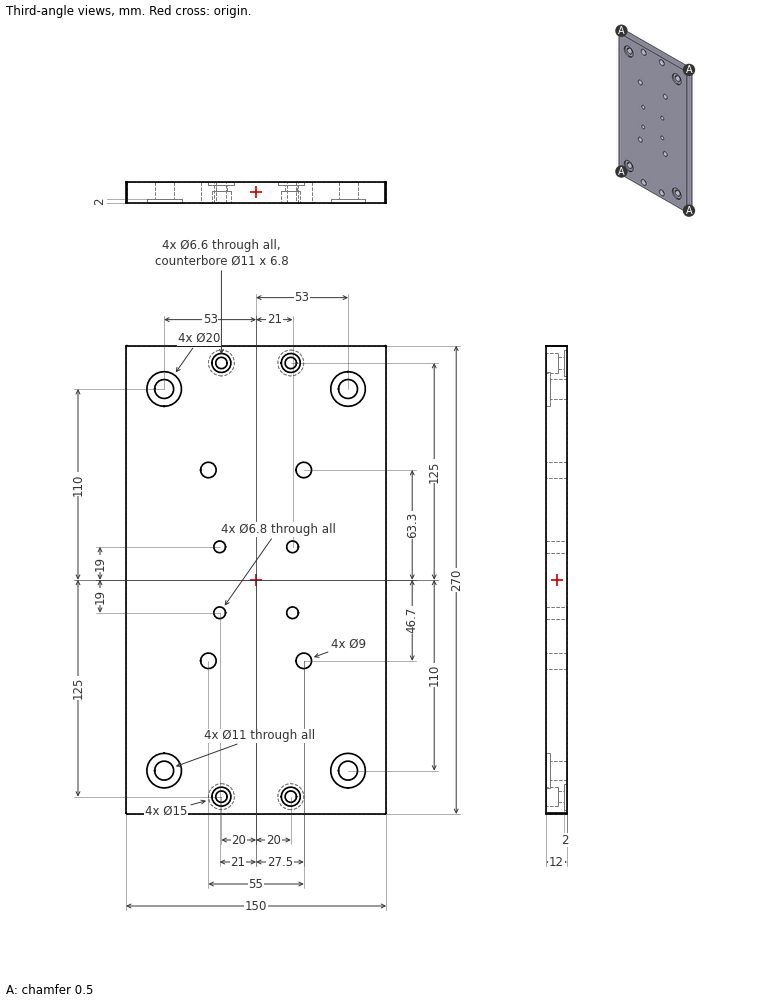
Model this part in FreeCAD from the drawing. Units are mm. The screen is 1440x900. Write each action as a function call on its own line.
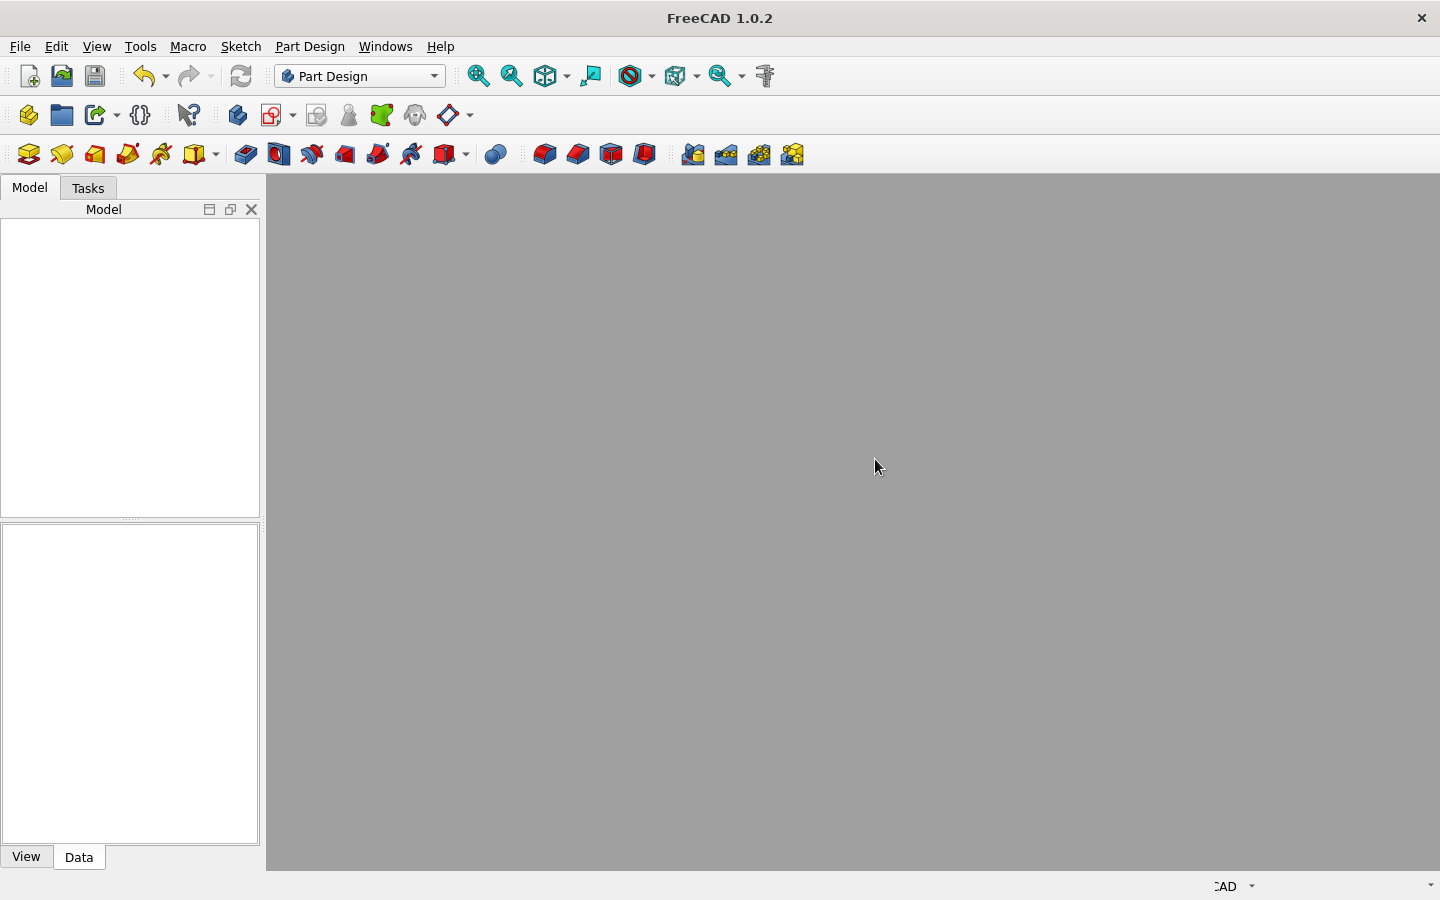
key(ctrl+n)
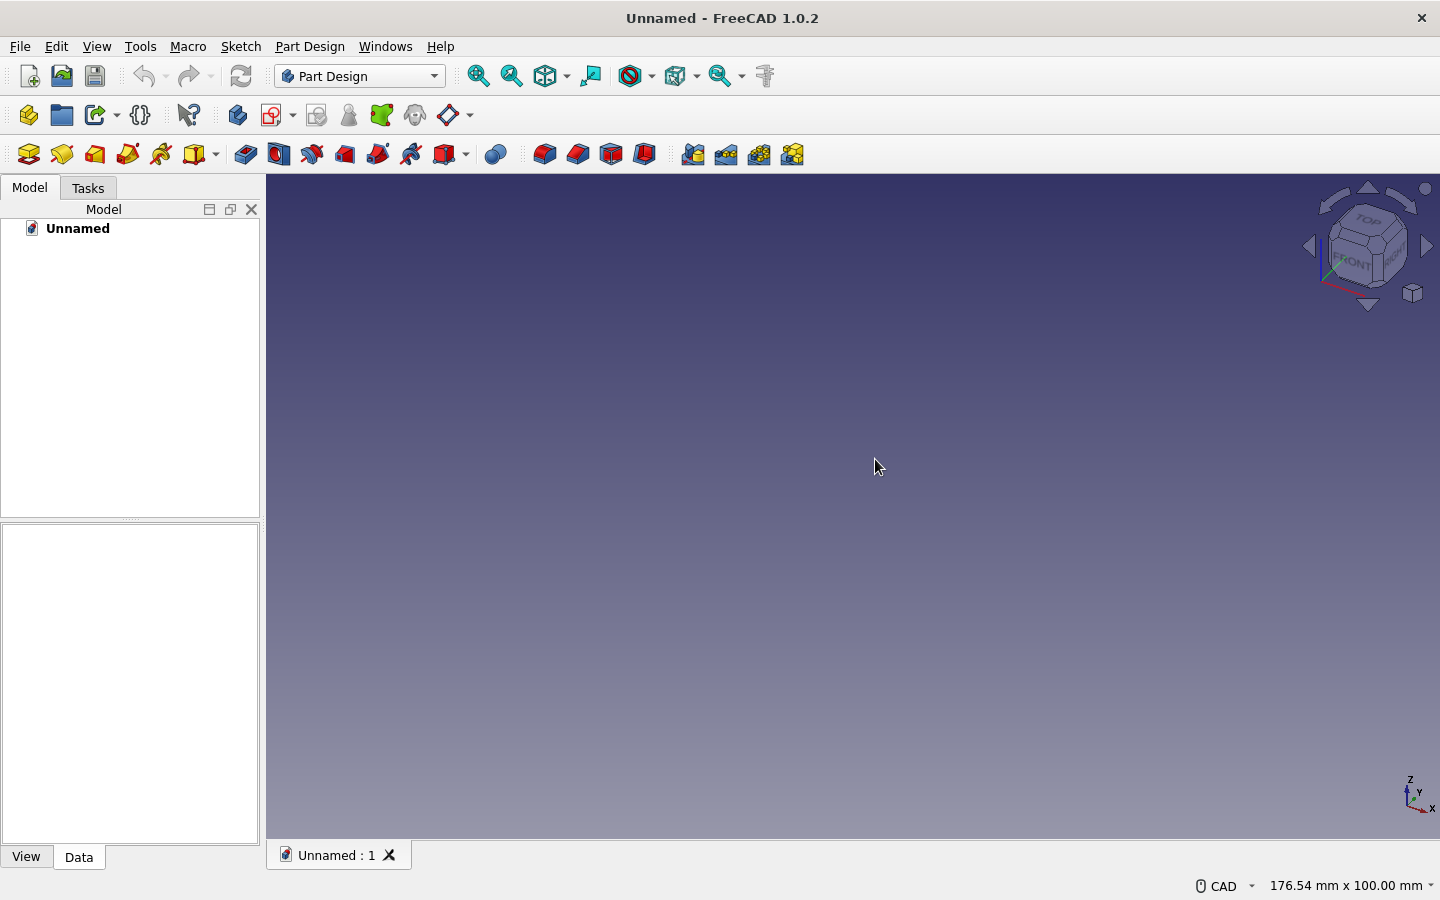
click(270, 116)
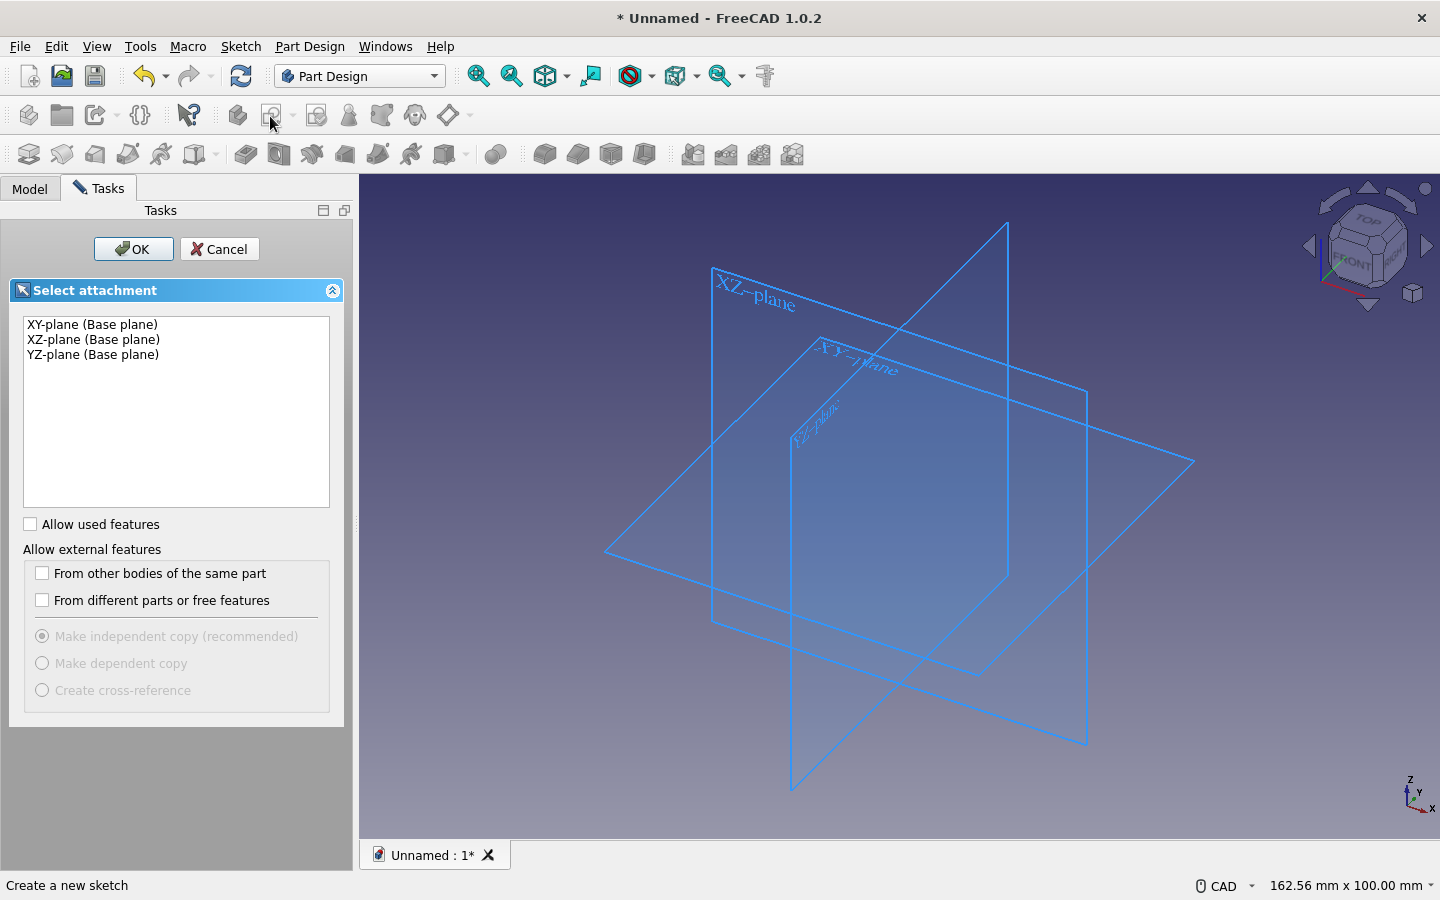
click(84, 340)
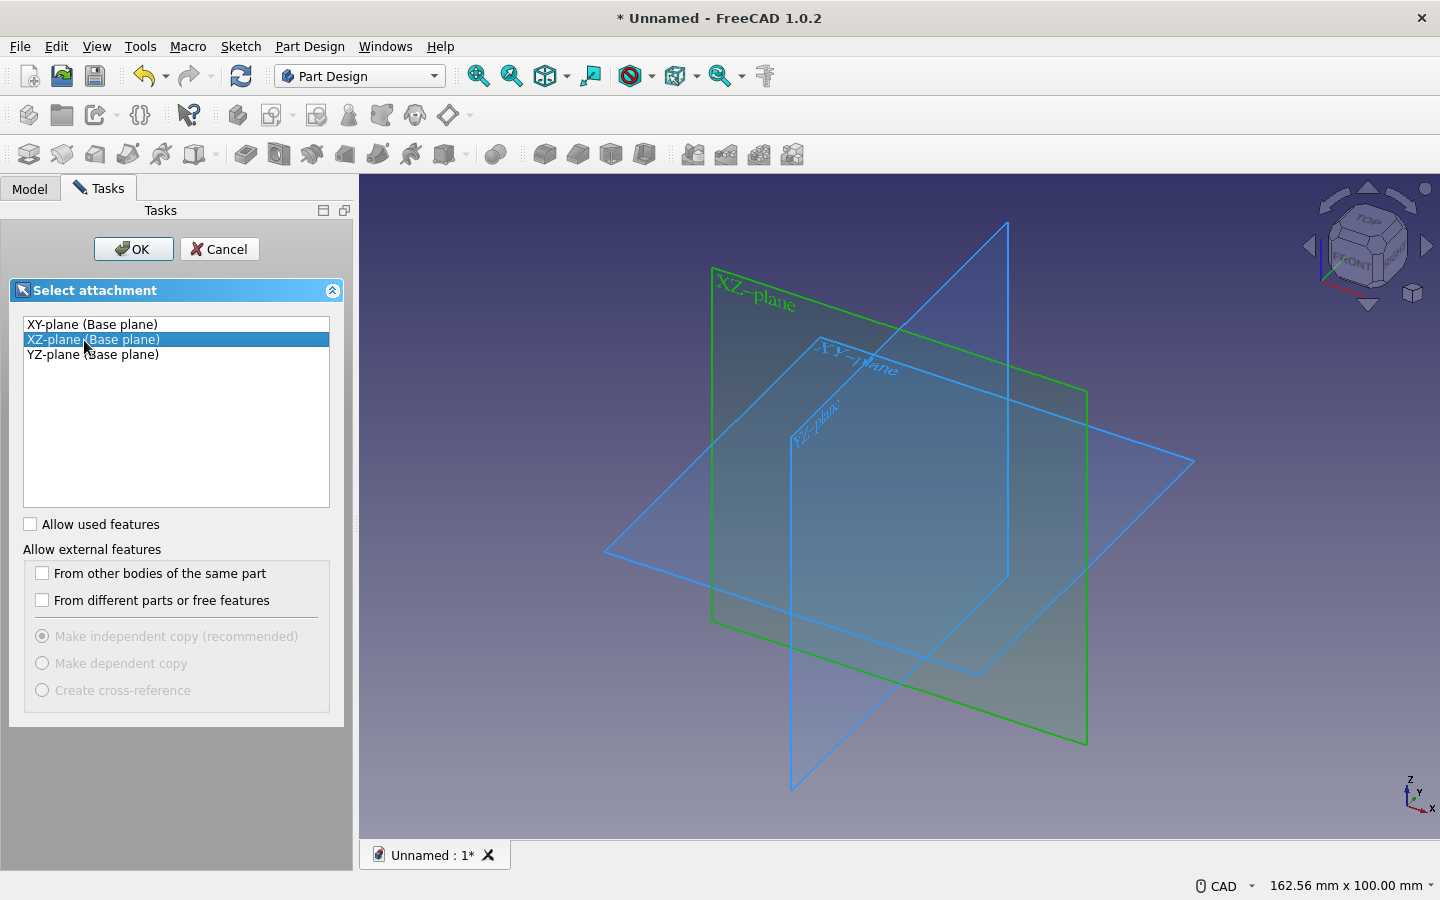
click(134, 249)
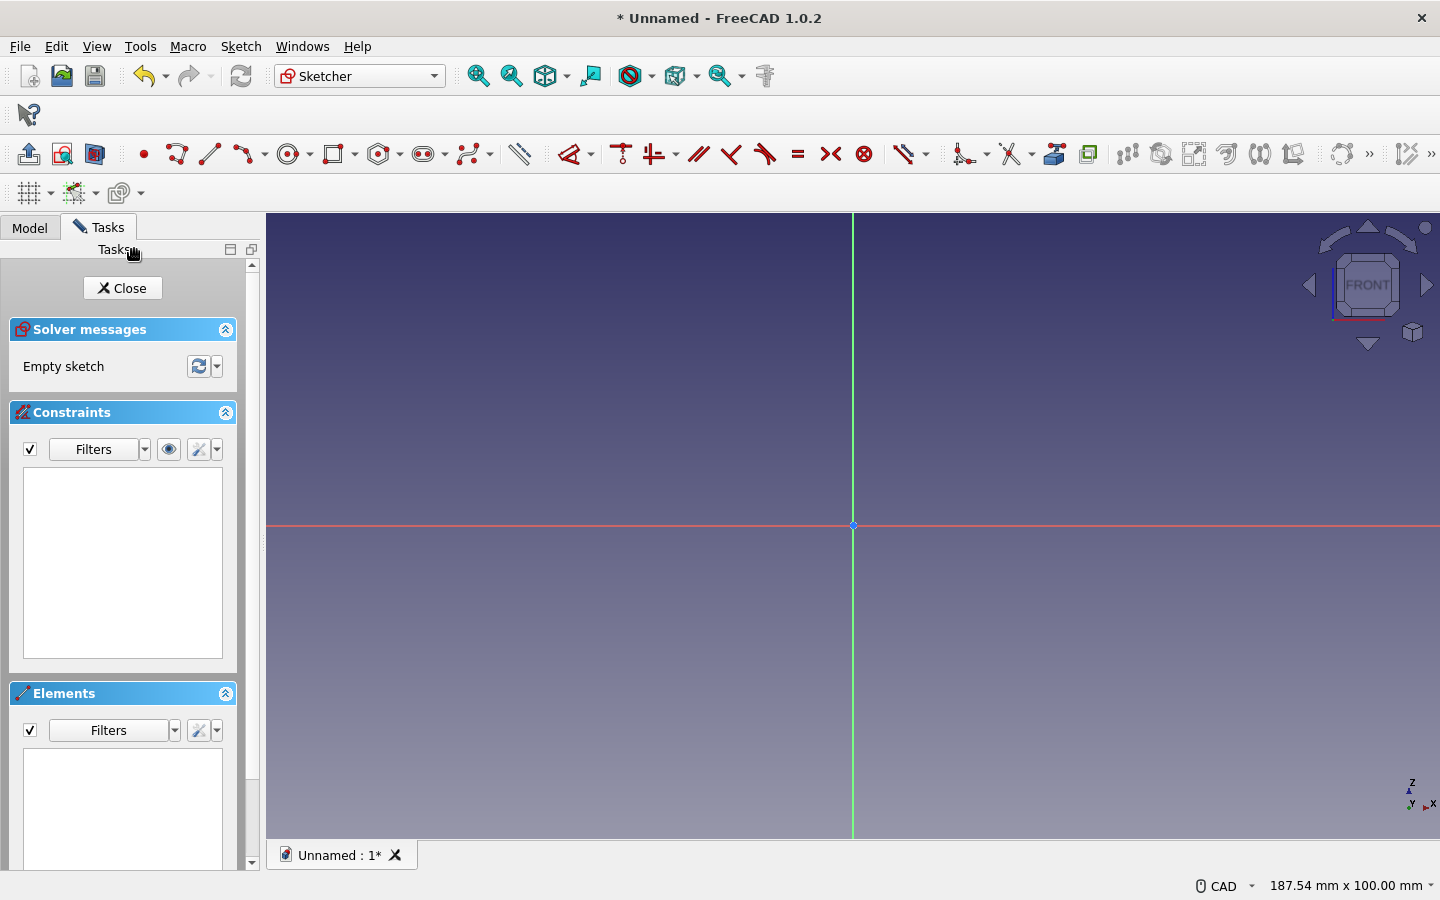
scroll(762, 526, down, 7)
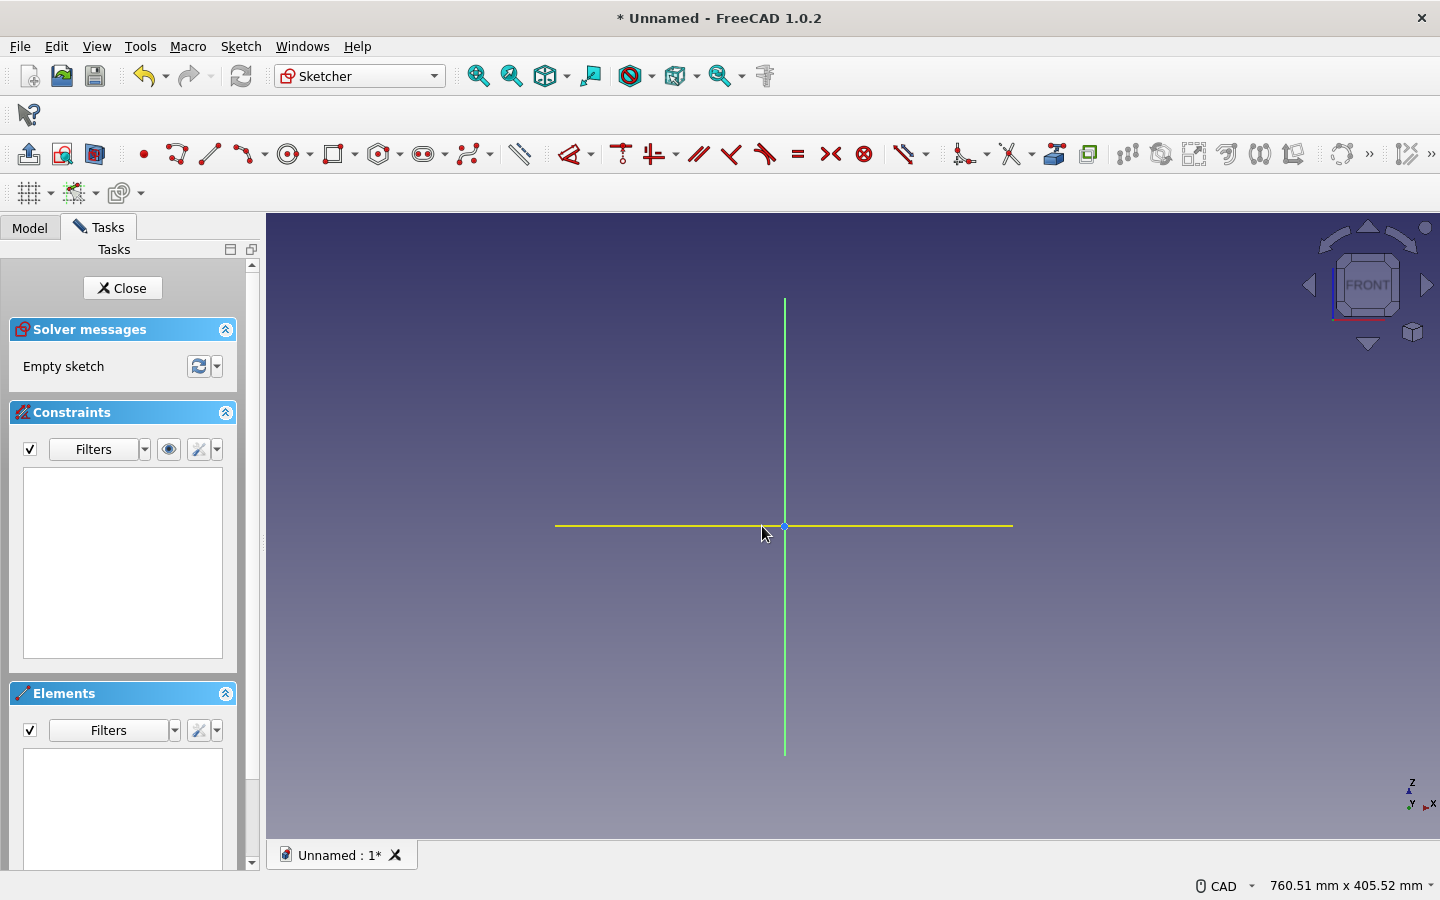
key(g)
key(v)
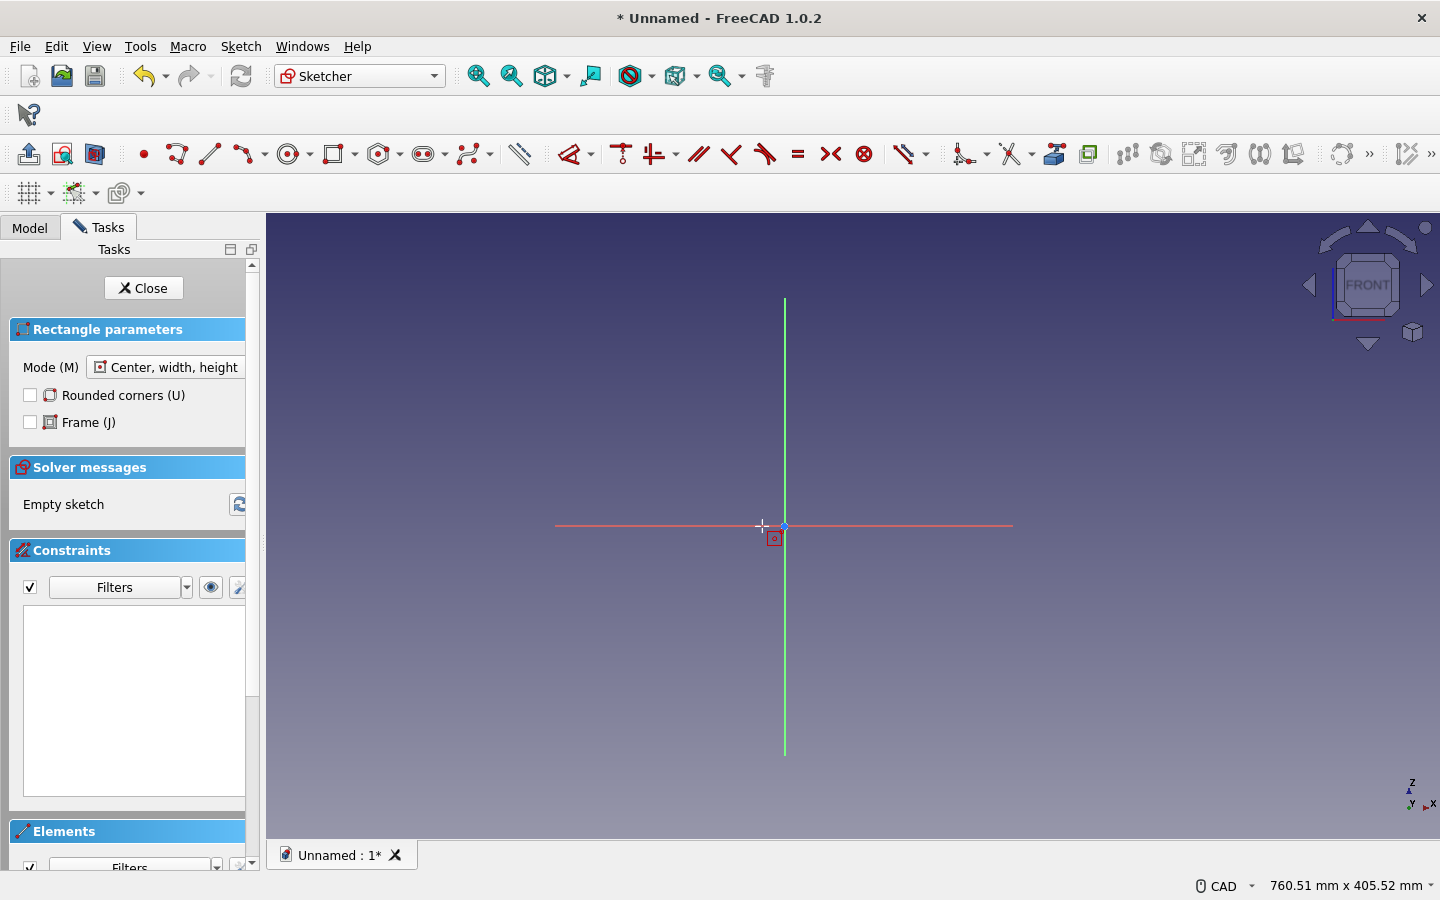
click(785, 526)
click(901, 318)
key(Escape)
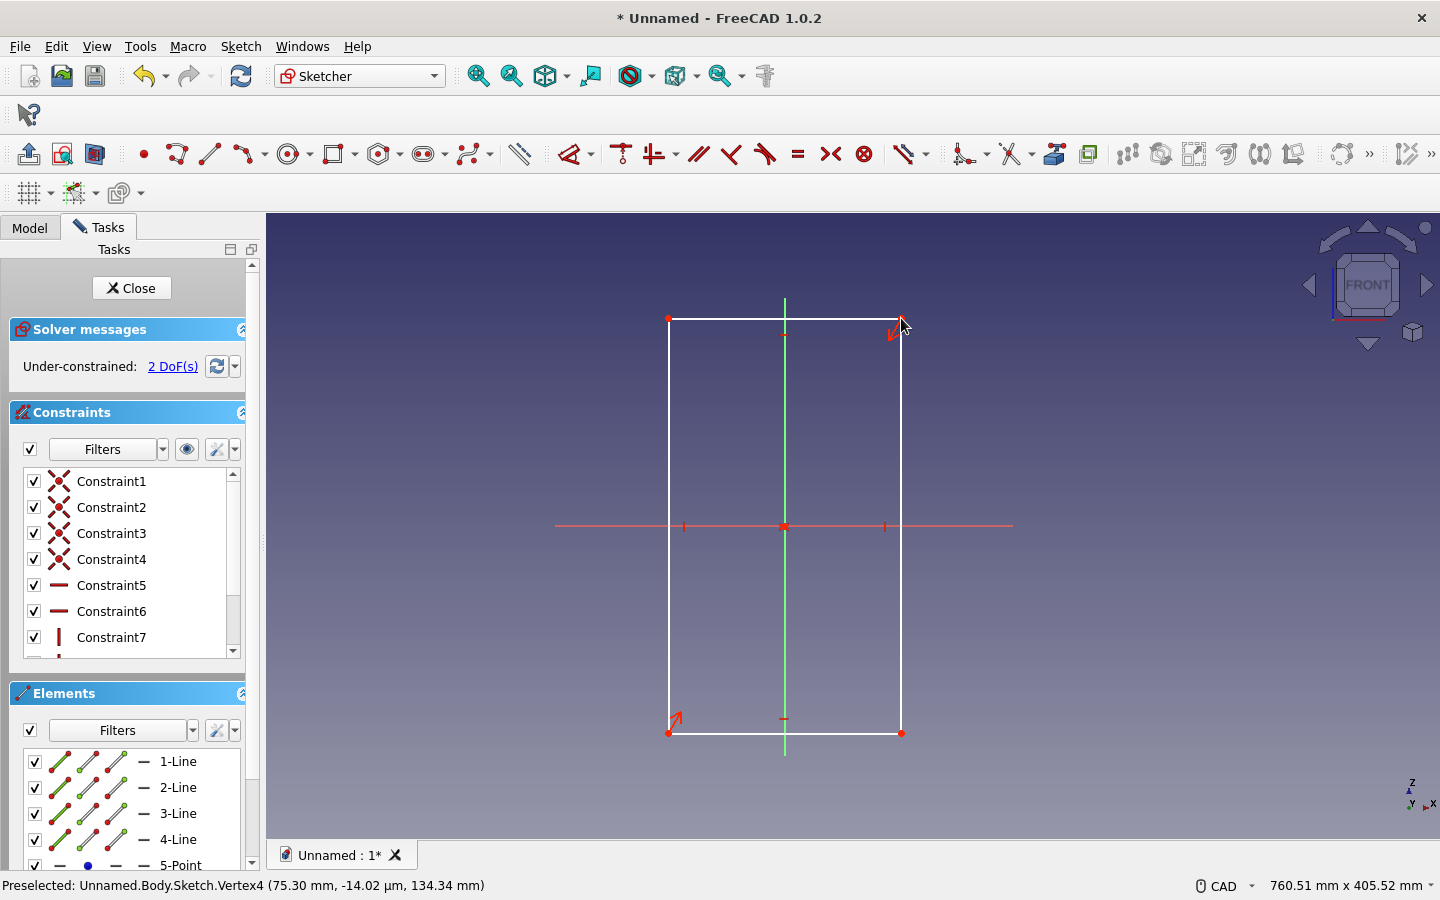
click(738, 734)